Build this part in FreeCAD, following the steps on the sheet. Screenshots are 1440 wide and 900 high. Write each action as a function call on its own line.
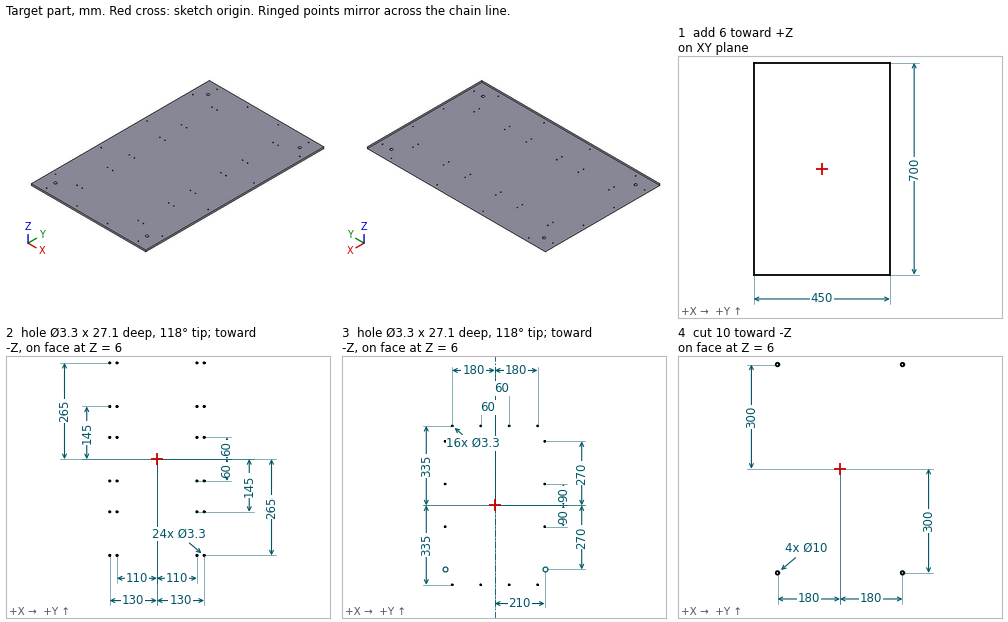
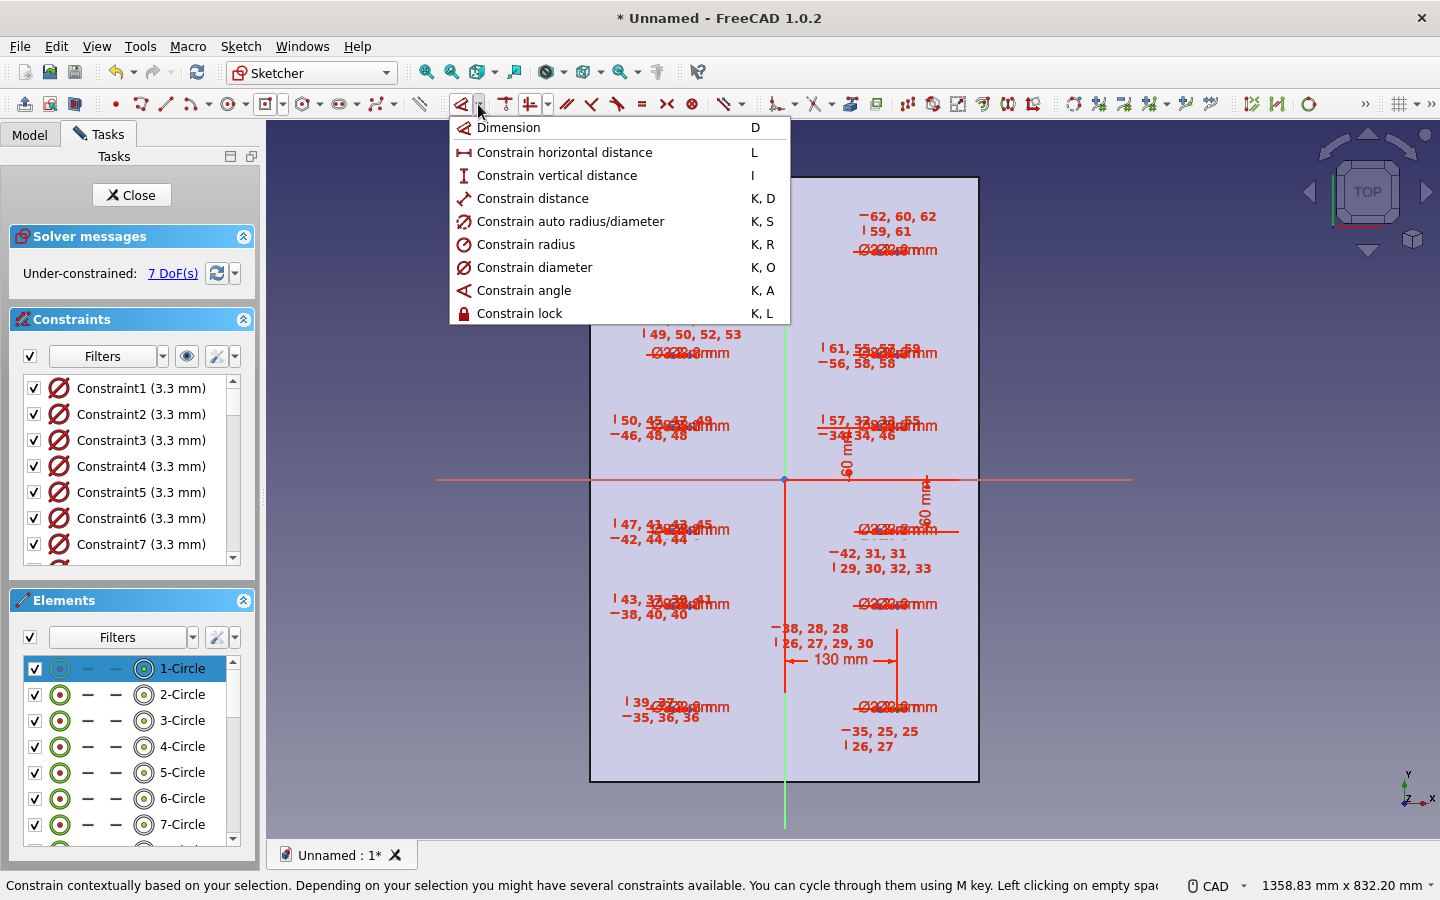
click(620, 176)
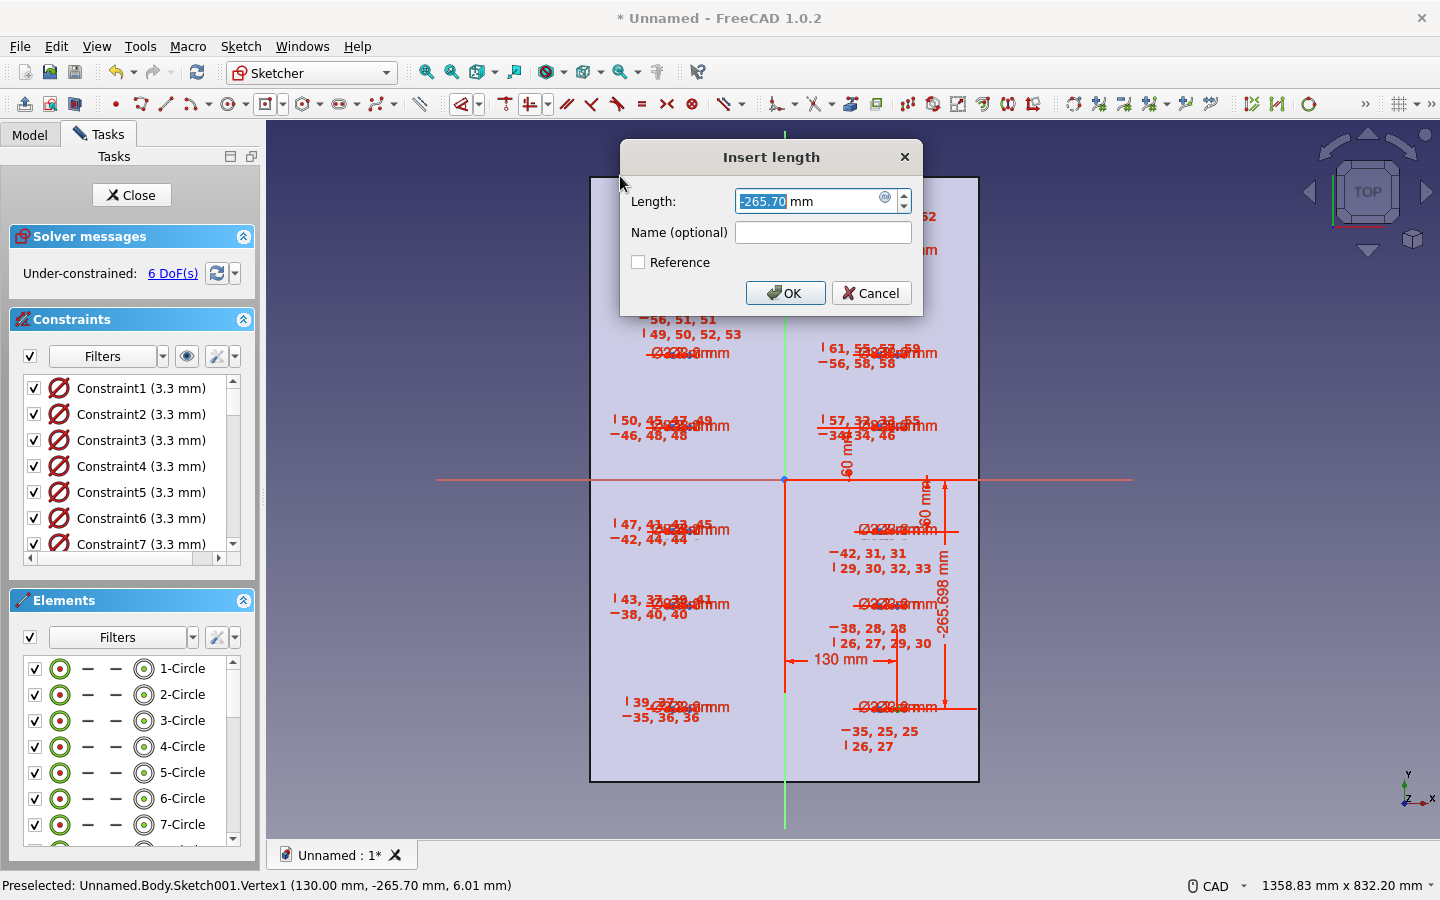
text(-265)
key(Return)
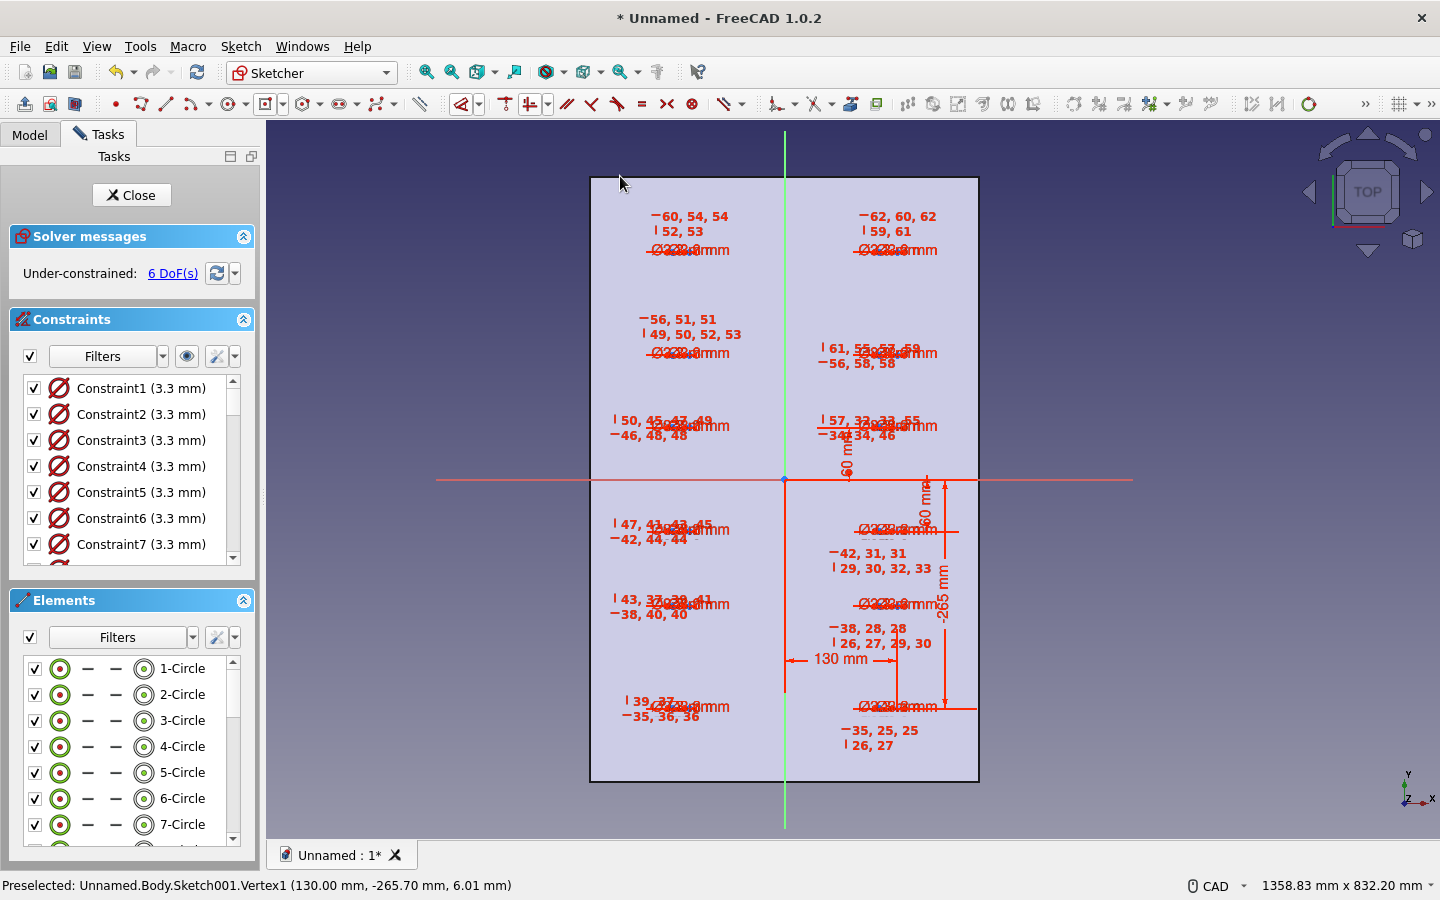
click(879, 709)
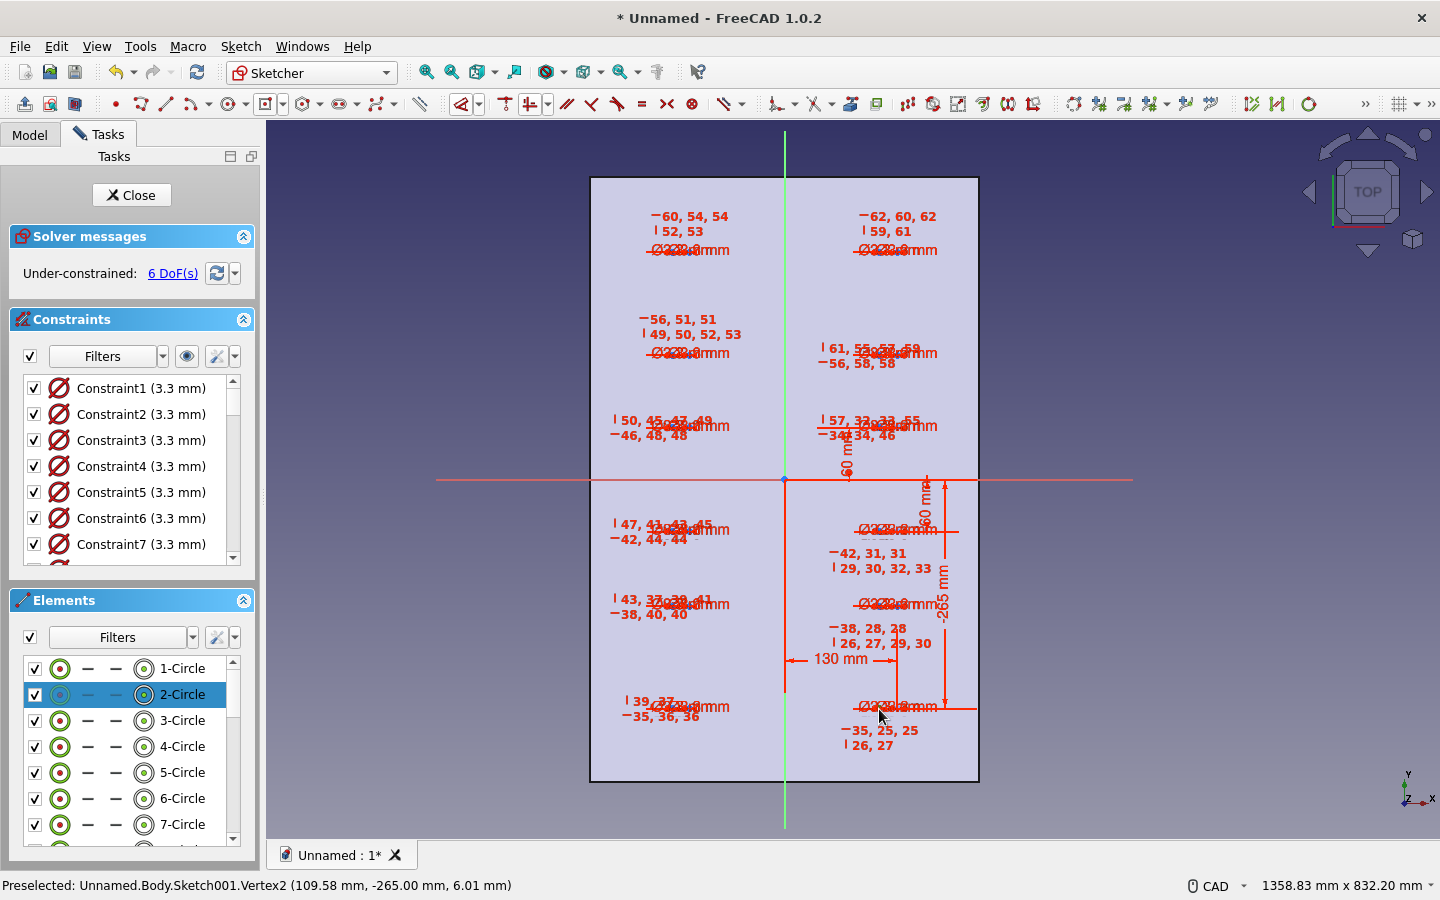
key(l)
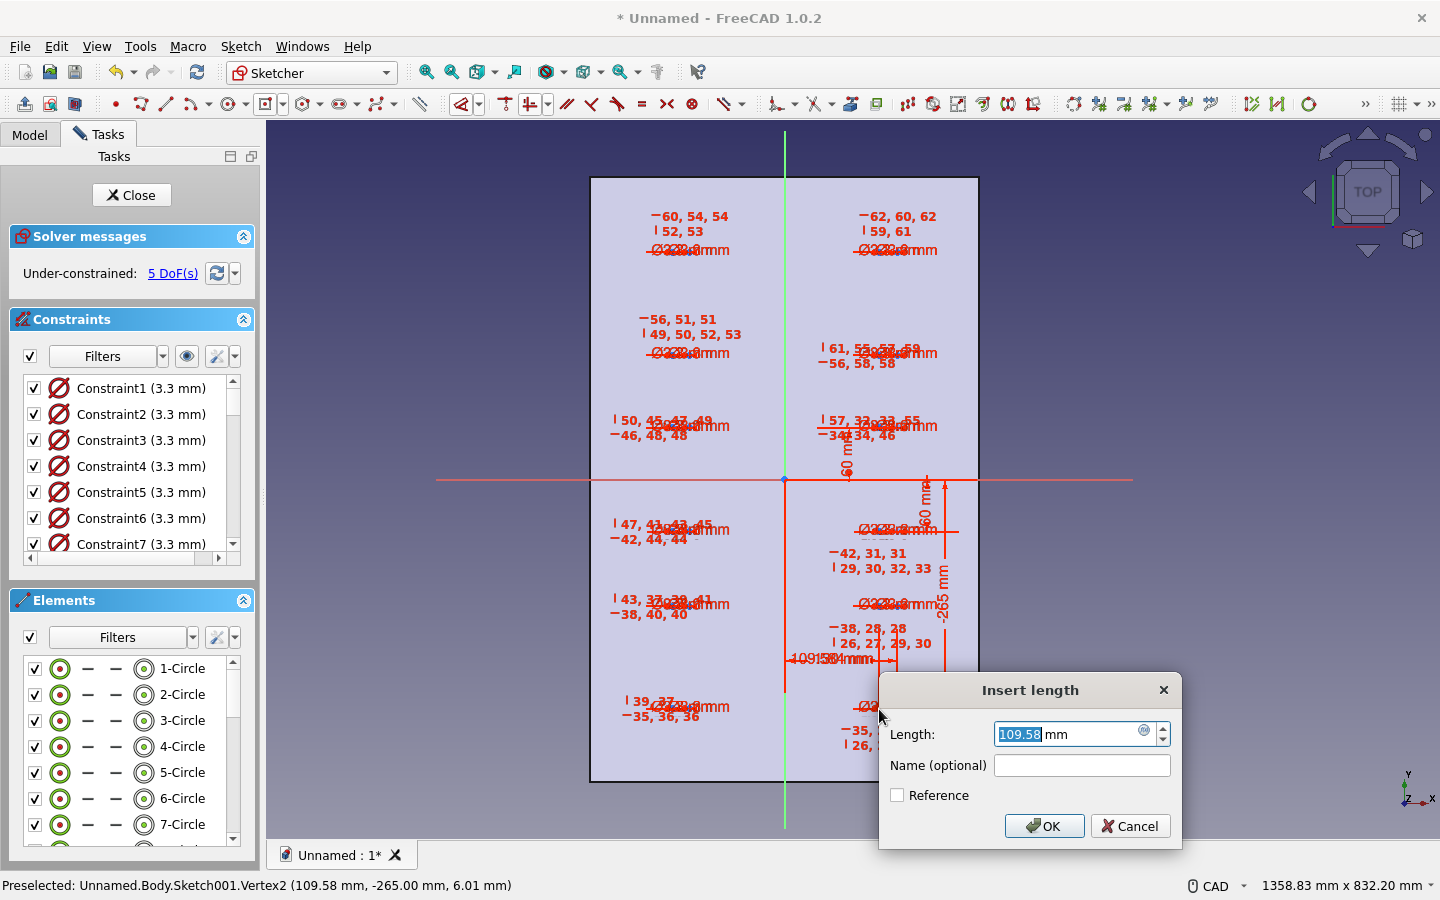
text(110)
key(Return)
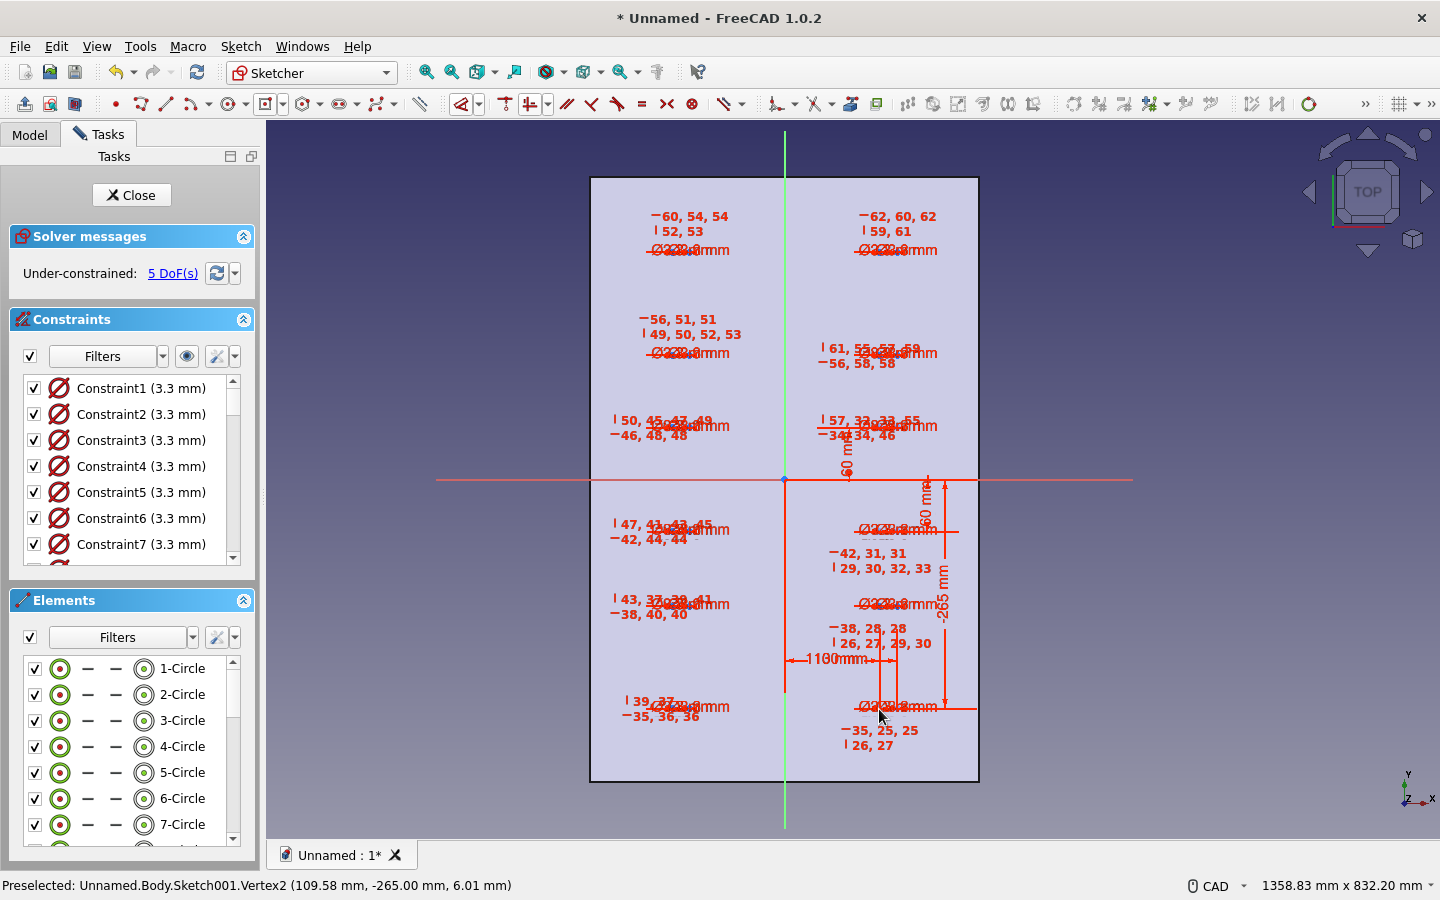
click(880, 606)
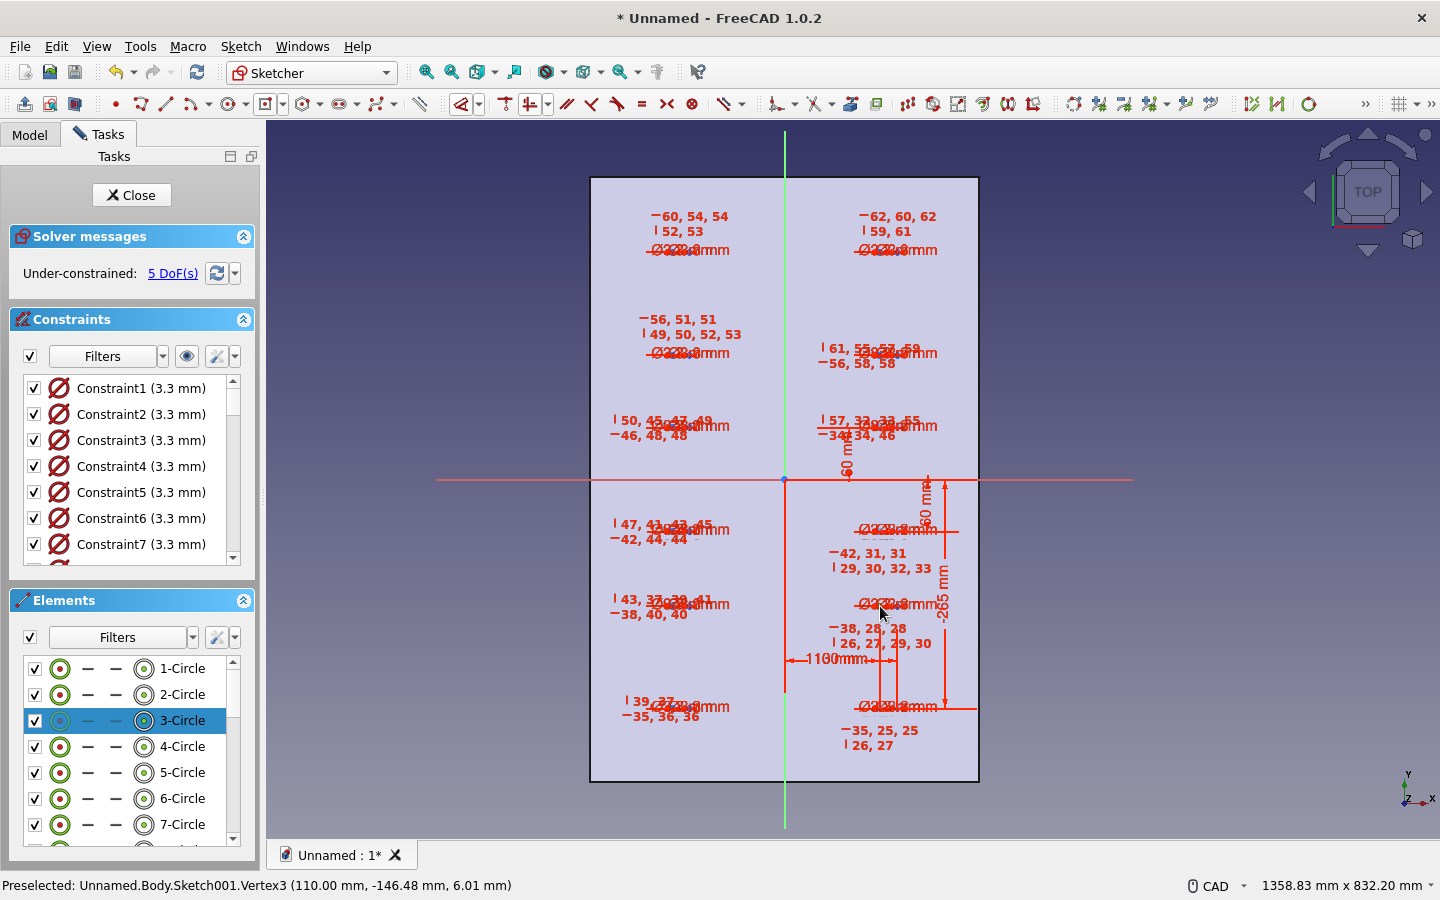
key(i)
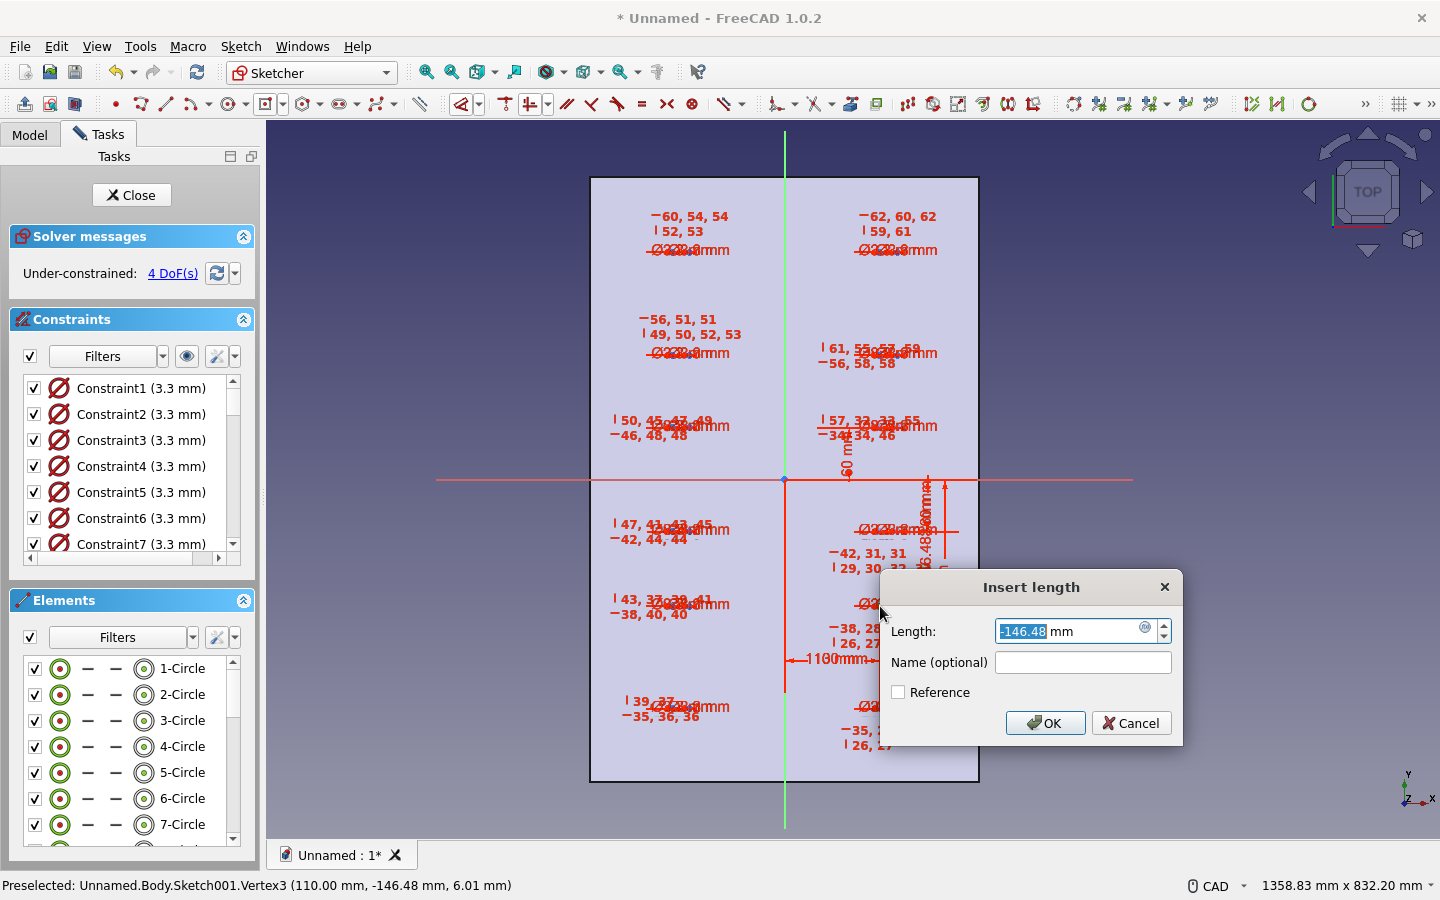
text(-145)
key(Return)